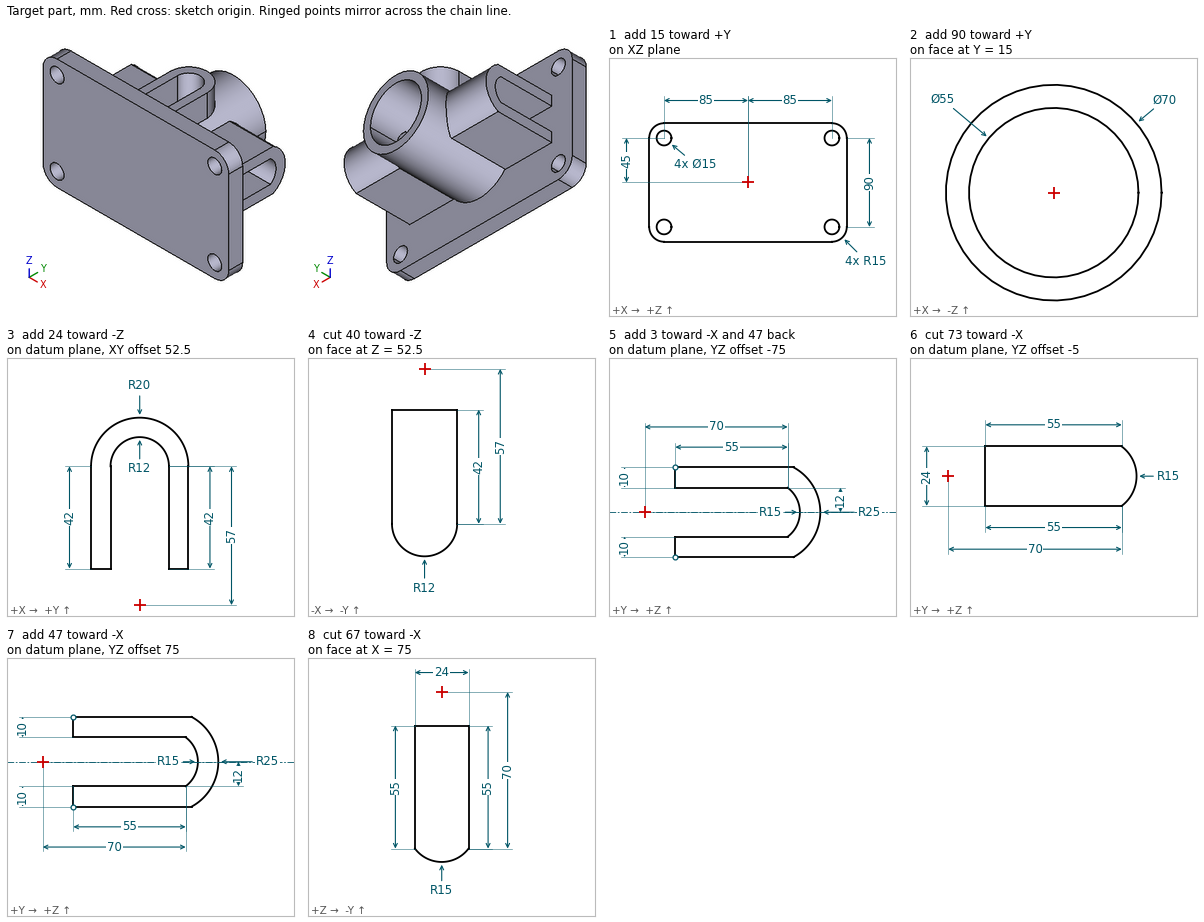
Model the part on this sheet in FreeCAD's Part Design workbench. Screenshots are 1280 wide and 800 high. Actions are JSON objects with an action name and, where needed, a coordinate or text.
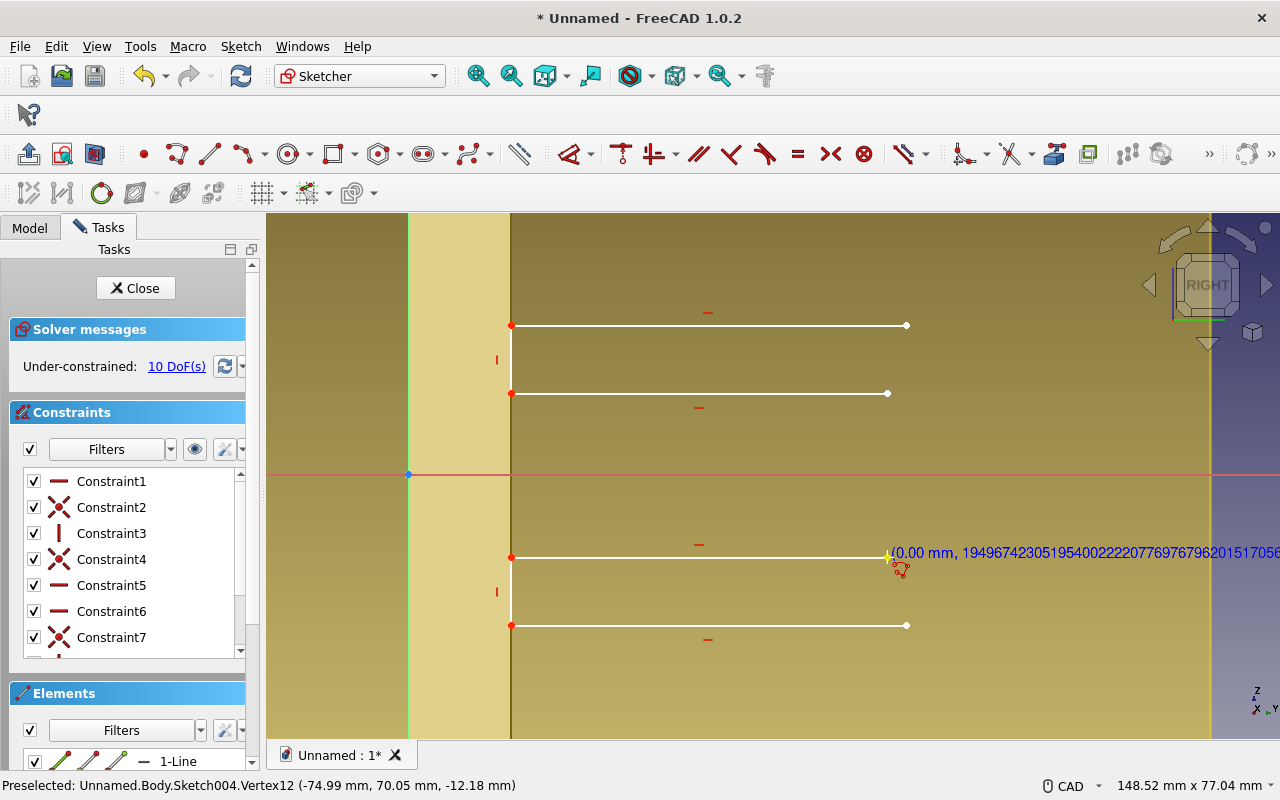
{"action": "key", "text": "g 3 a"}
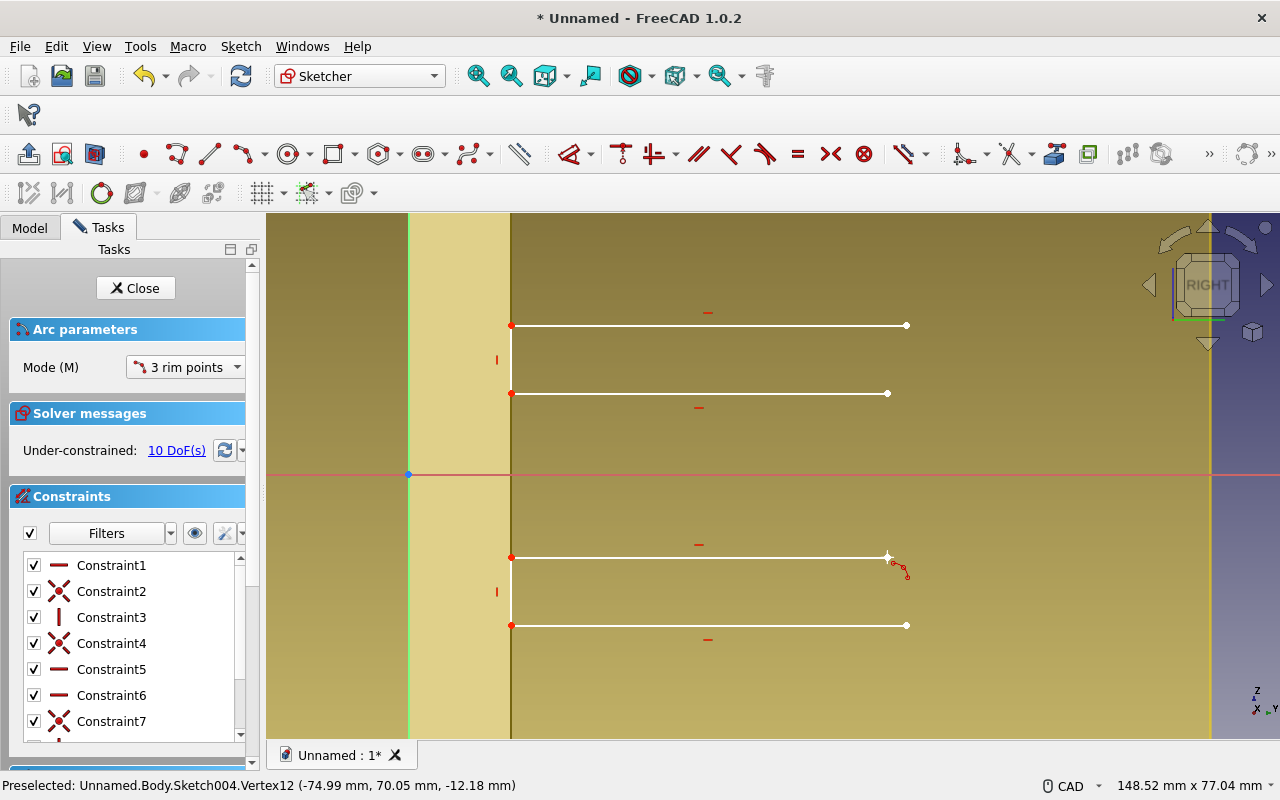
{"action": "left_click", "coordinate": [906, 326]}
{"action": "left_click", "coordinate": [906, 626]}
{"action": "left_click", "coordinate": [992, 511]}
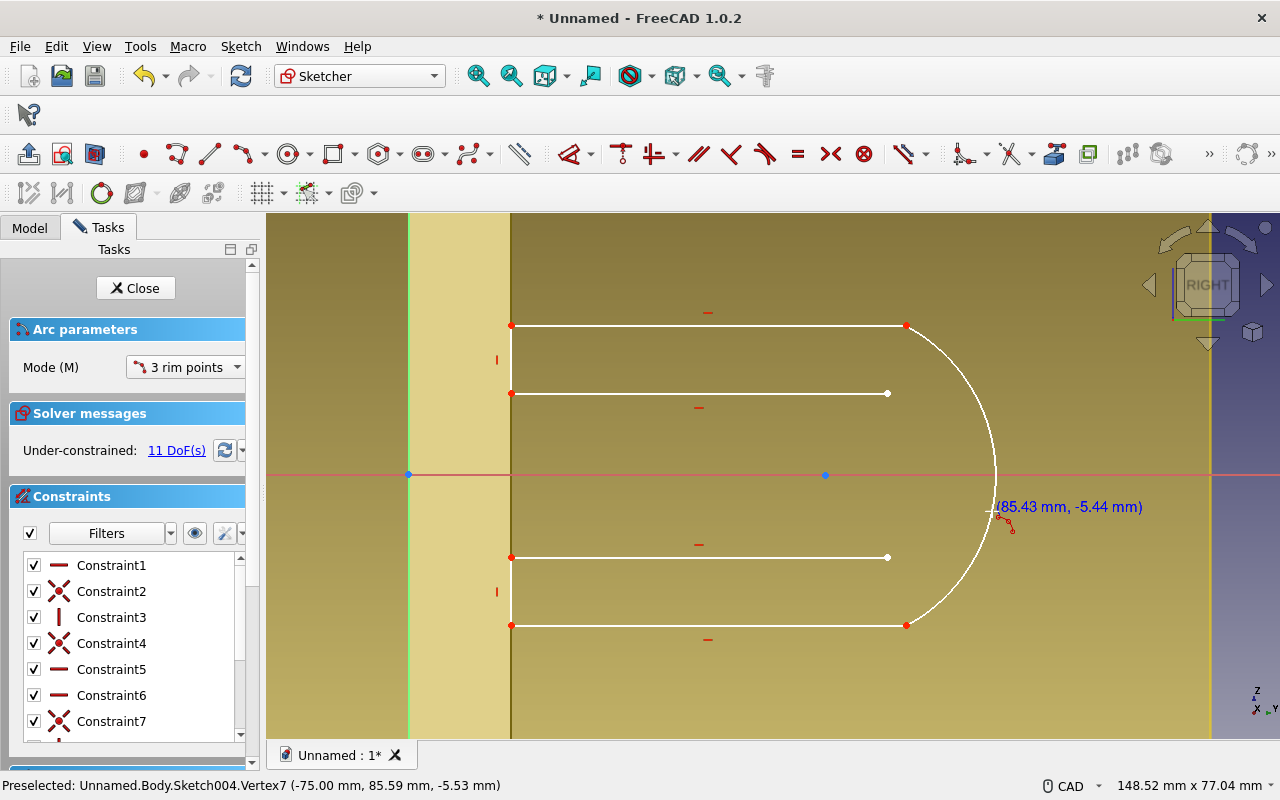
{"action": "left_click", "coordinate": [887, 558]}
{"action": "left_click", "coordinate": [887, 394]}
{"action": "left_click", "coordinate": [926, 494]}
{"action": "key", "text": "Escape"}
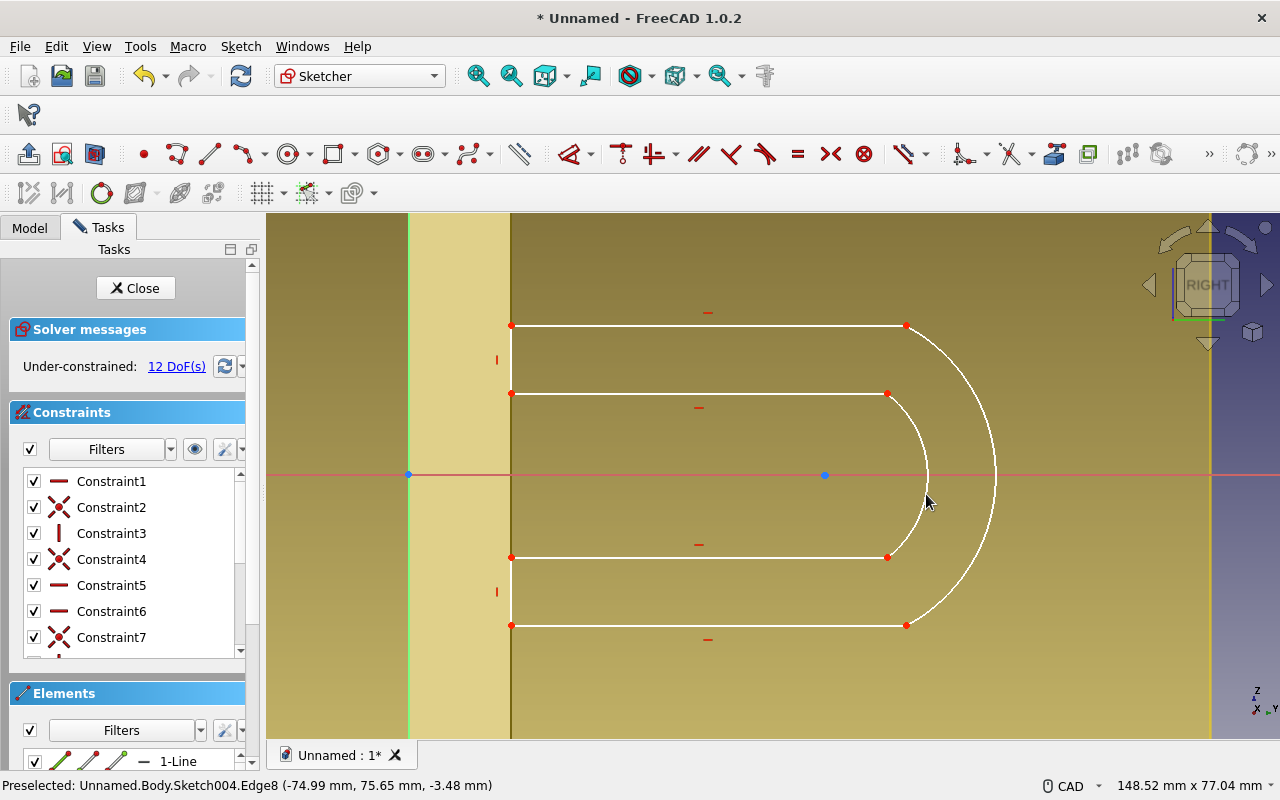
{"action": "left_click", "coordinate": [980, 547]}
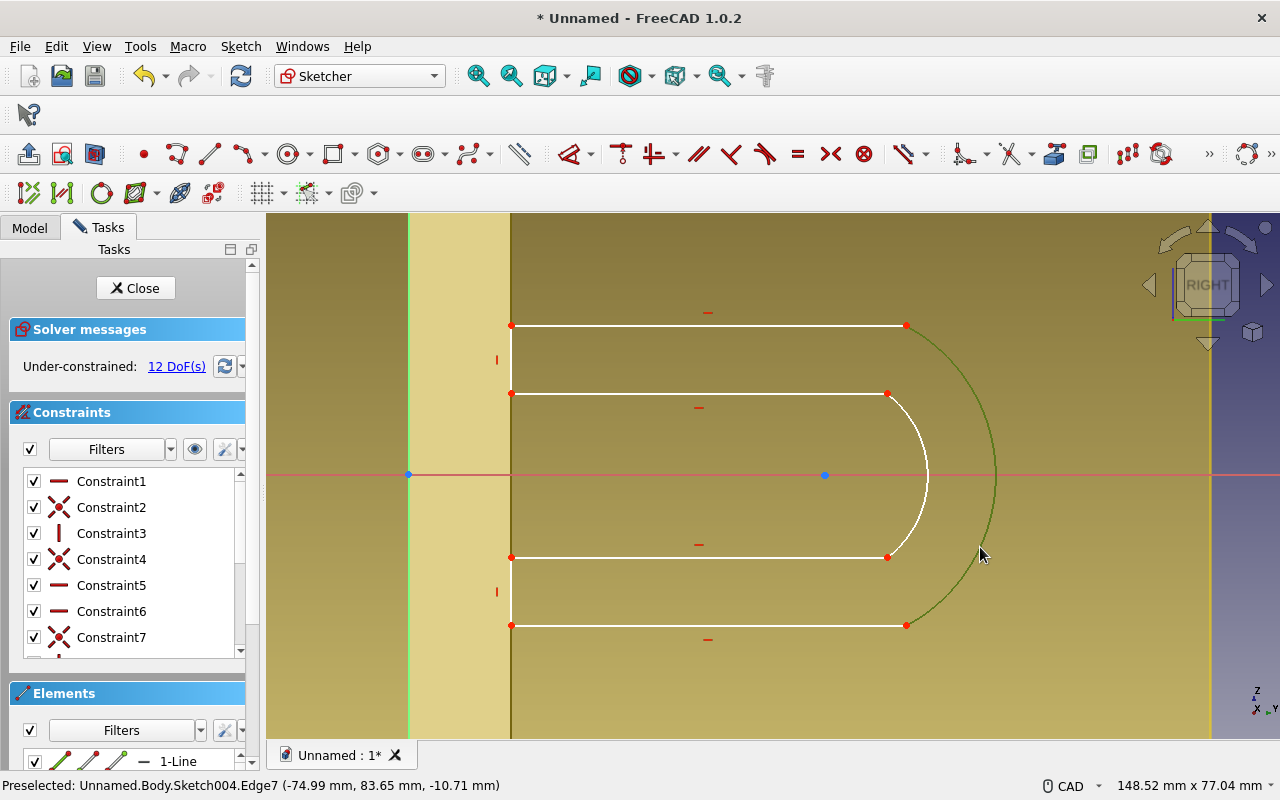
{"action": "left_click", "coordinate": [921, 513]}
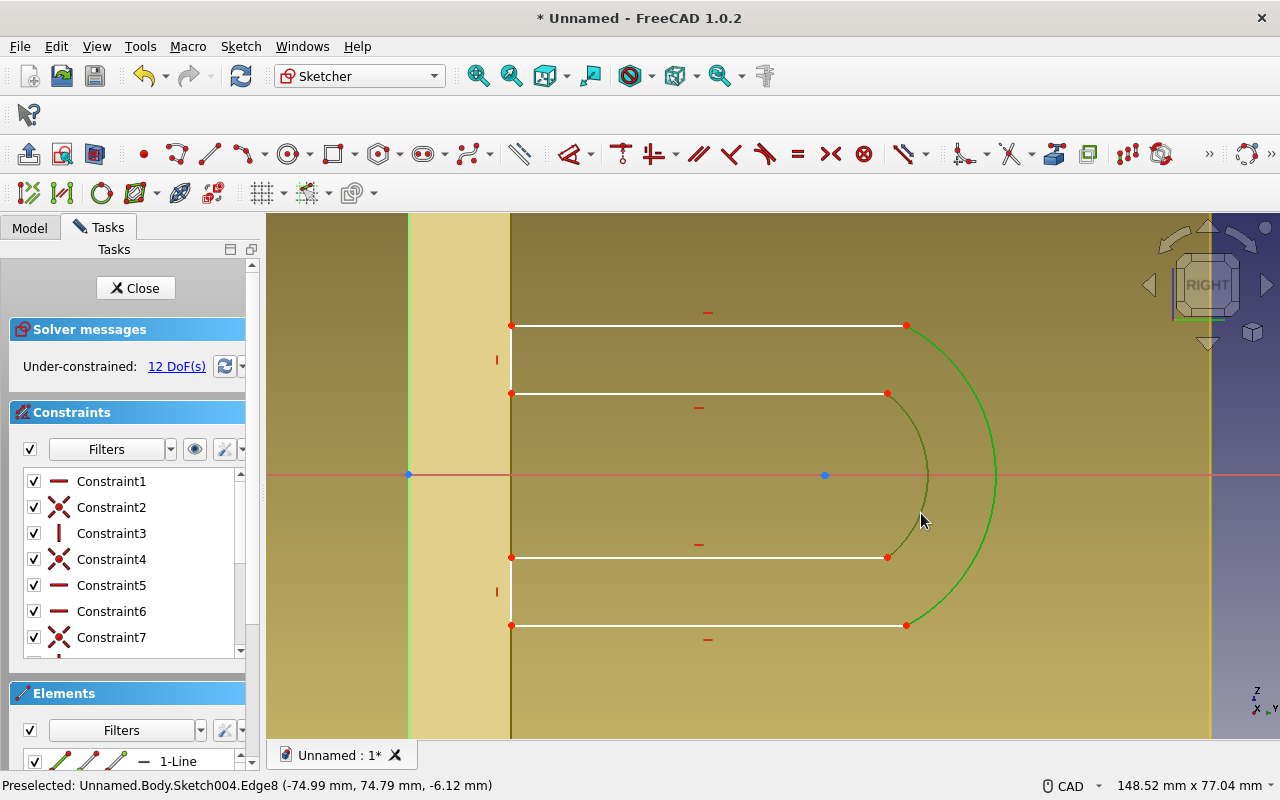
{"action": "key", "text": "c"}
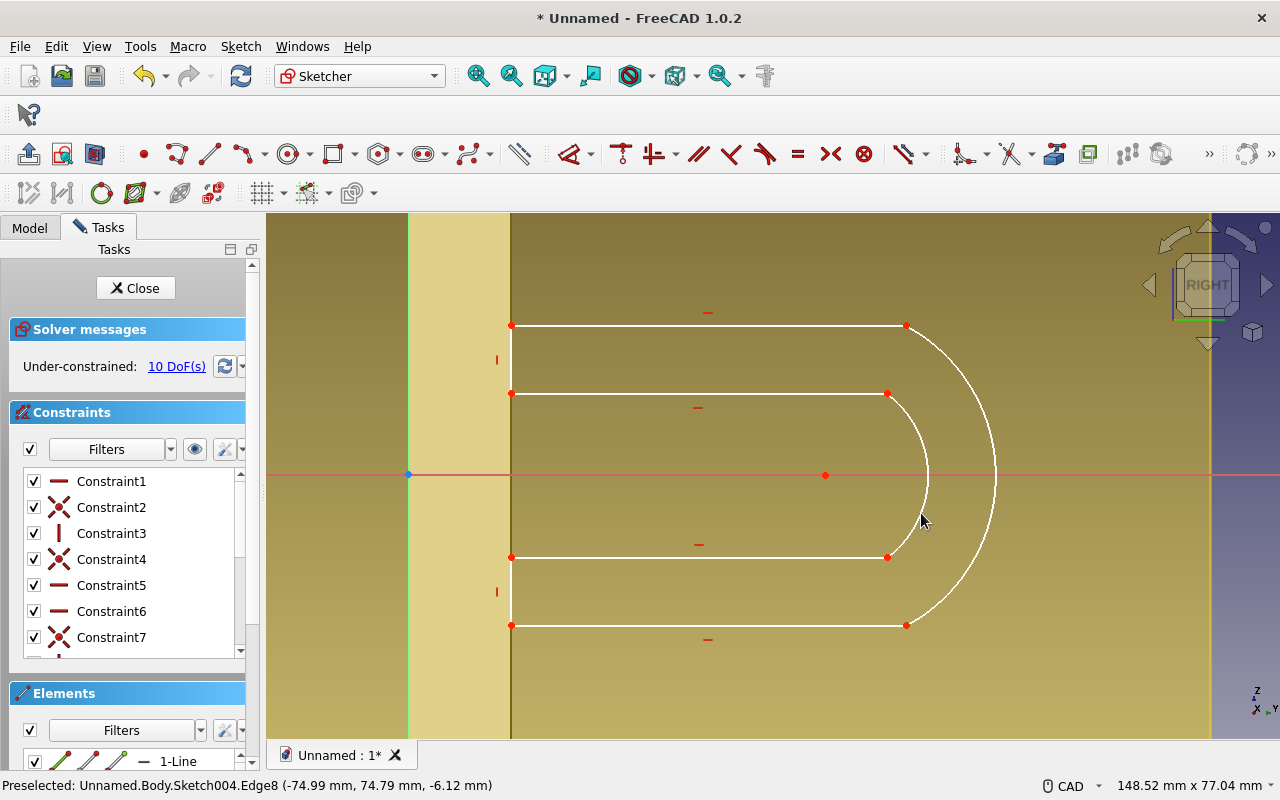
{"action": "left_click", "coordinate": [826, 476]}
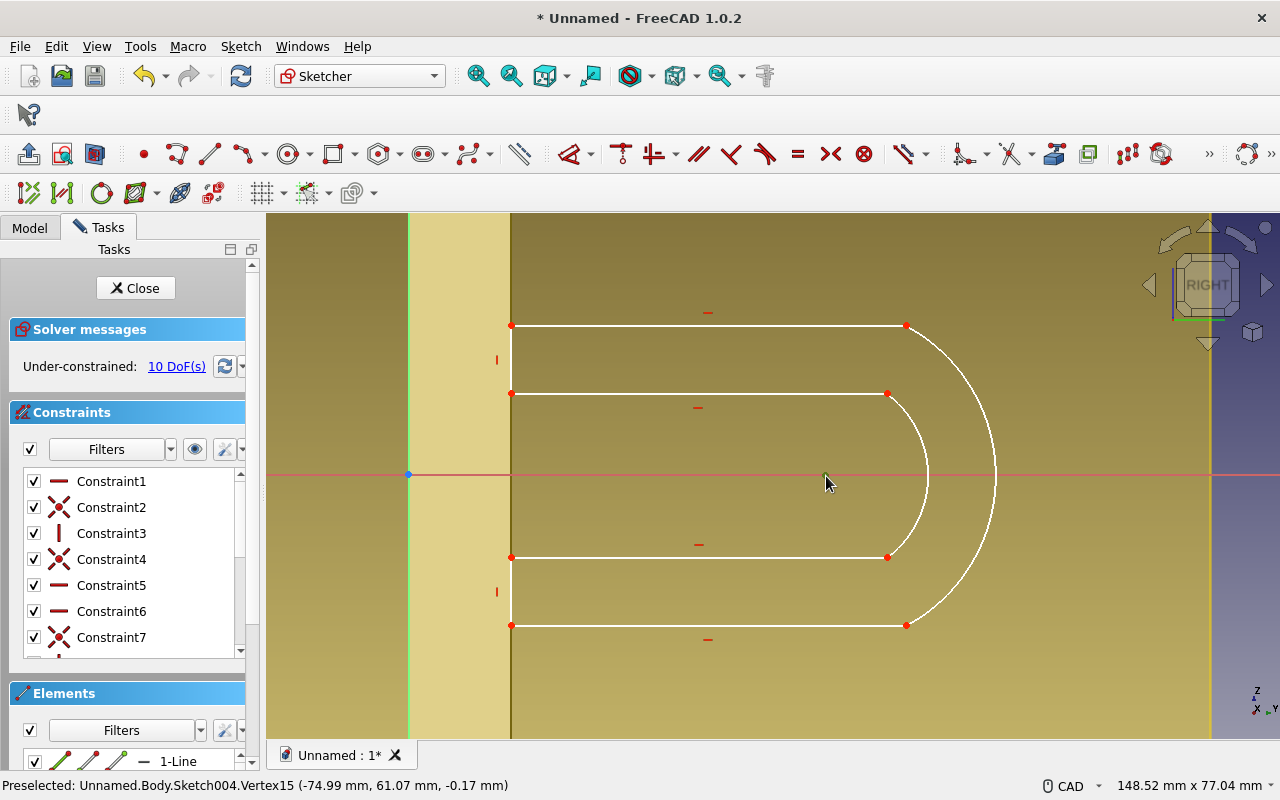
{"action": "left_click", "coordinate": [353, 475]}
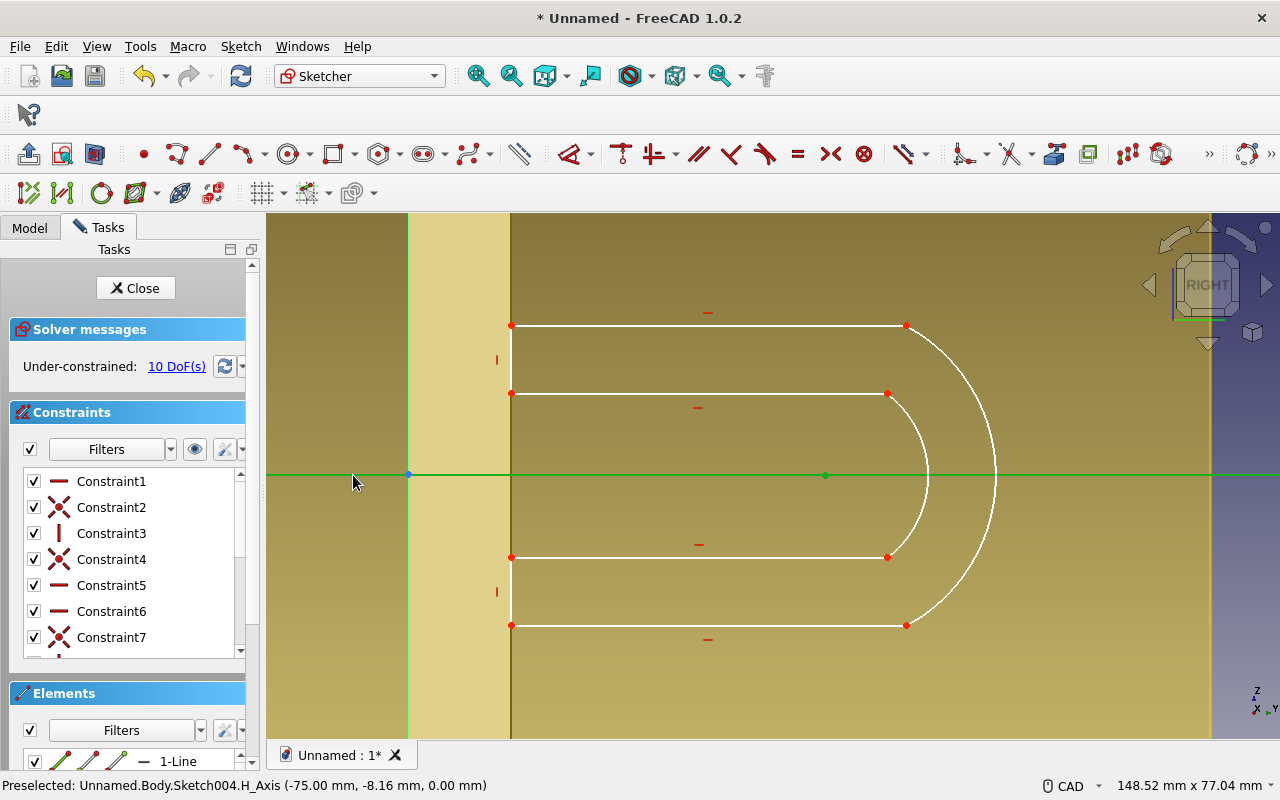
{"action": "key", "text": "c"}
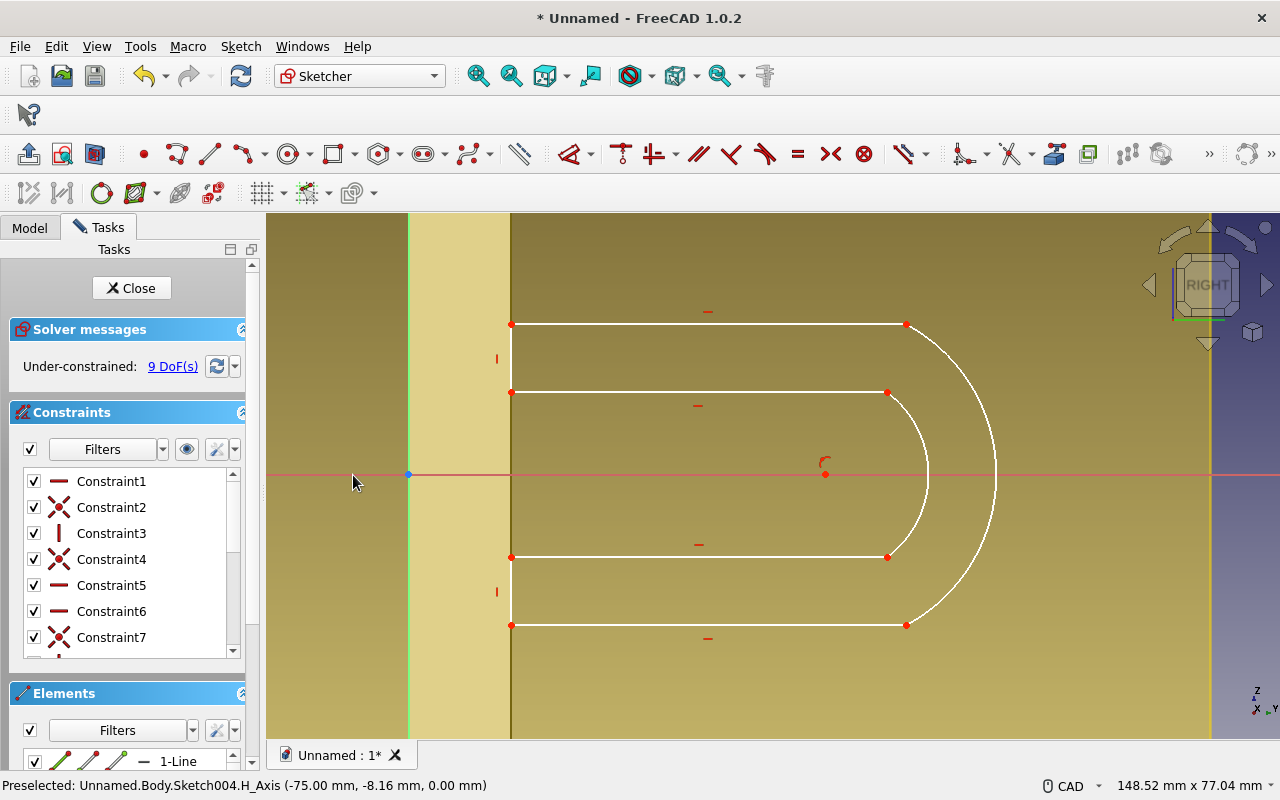
{"action": "left_click", "coordinate": [511, 324]}